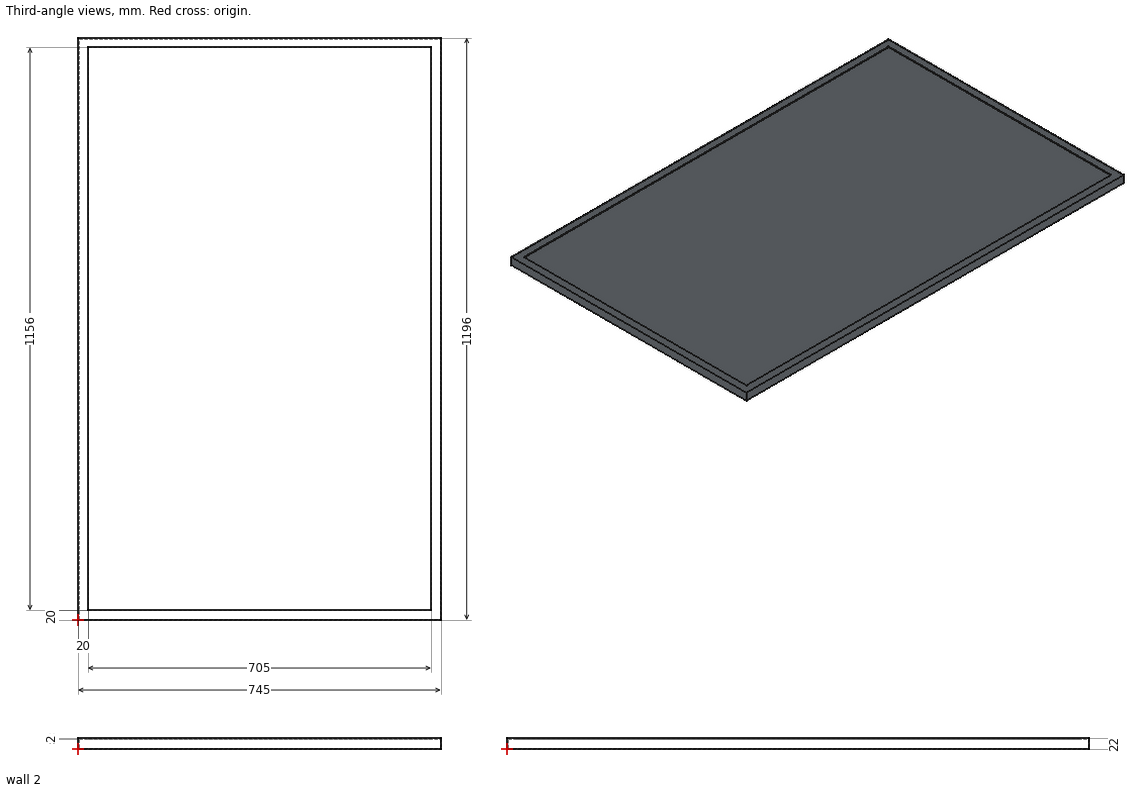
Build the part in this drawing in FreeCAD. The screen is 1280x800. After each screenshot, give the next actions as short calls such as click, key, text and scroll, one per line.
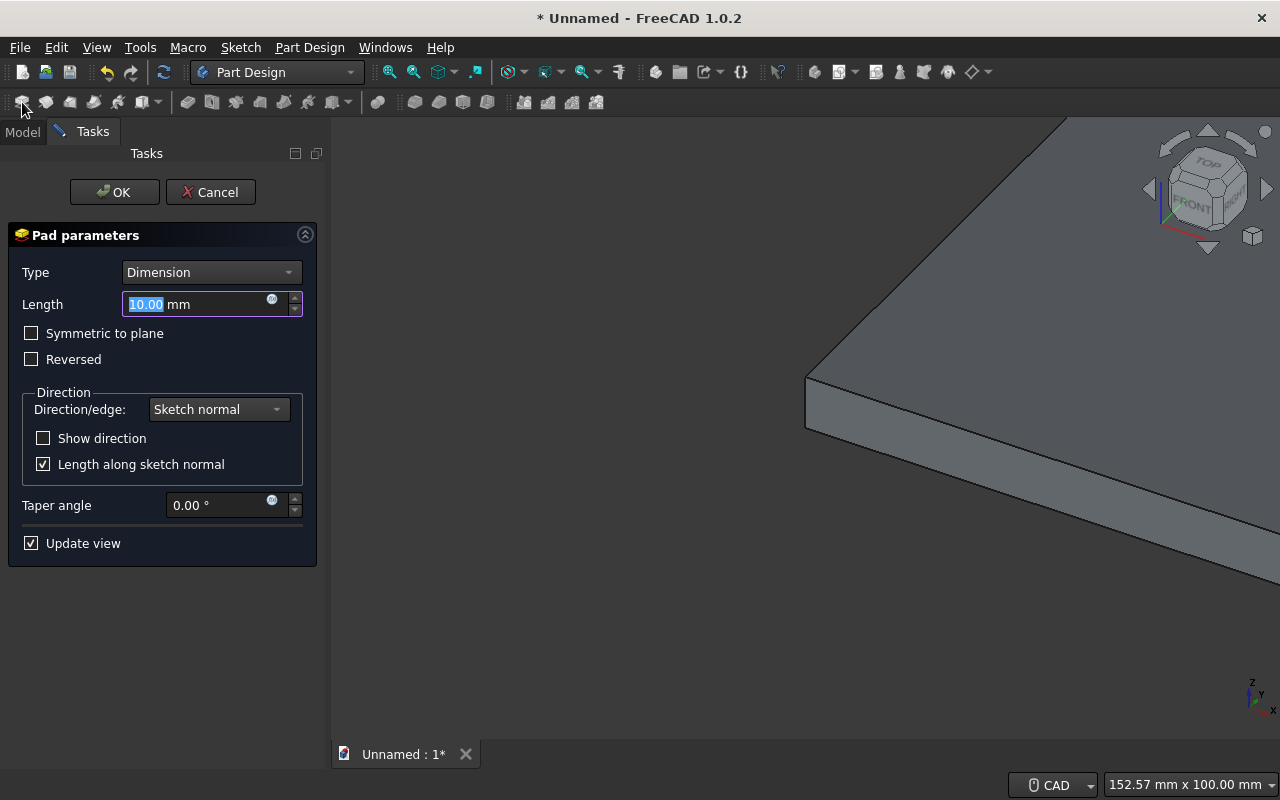
text(22)
key(Tab)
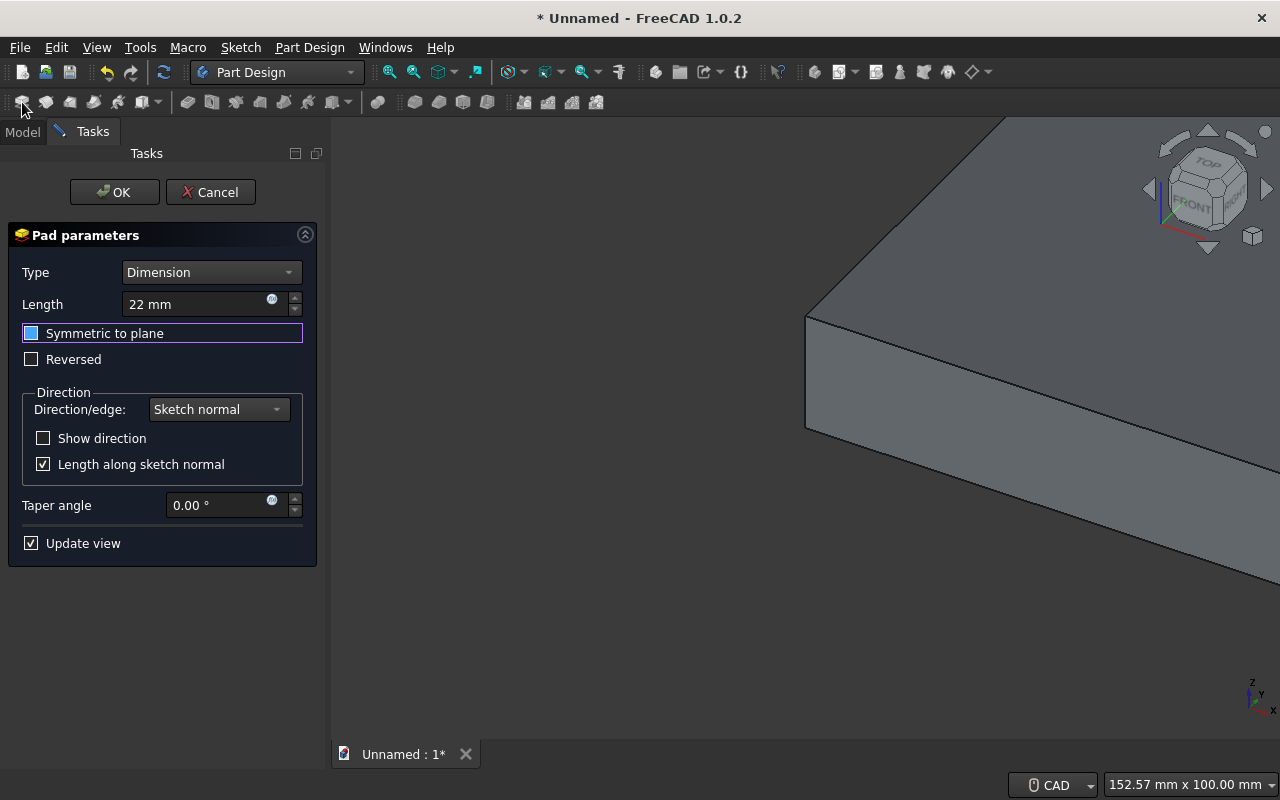
click(115, 192)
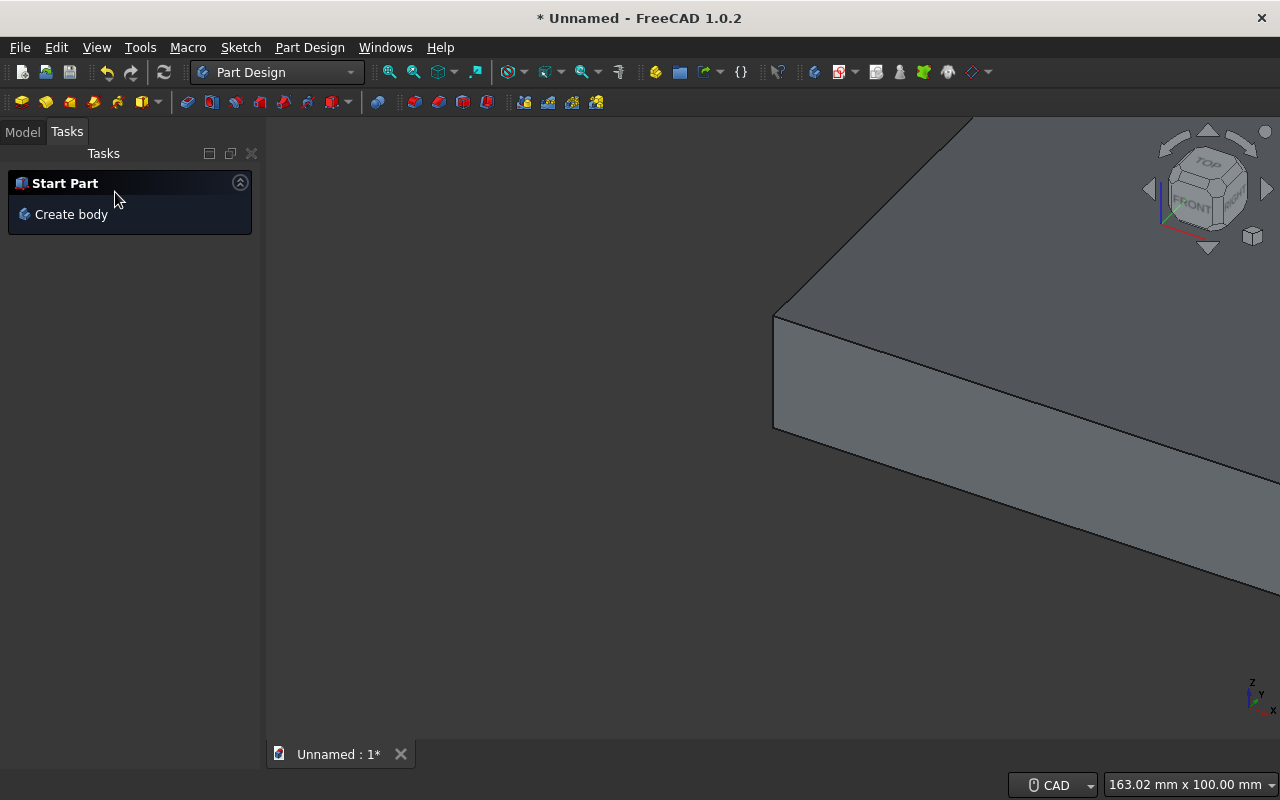
click(390, 72)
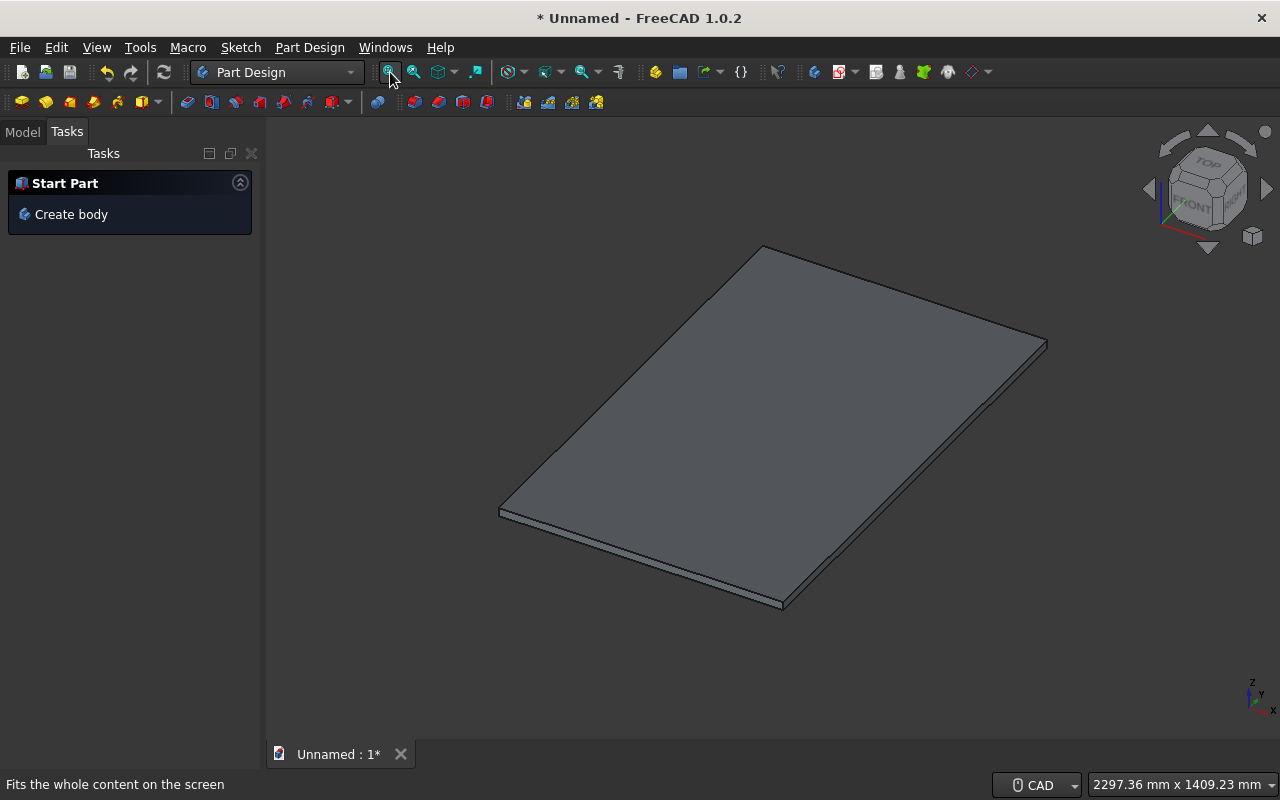
click(811, 386)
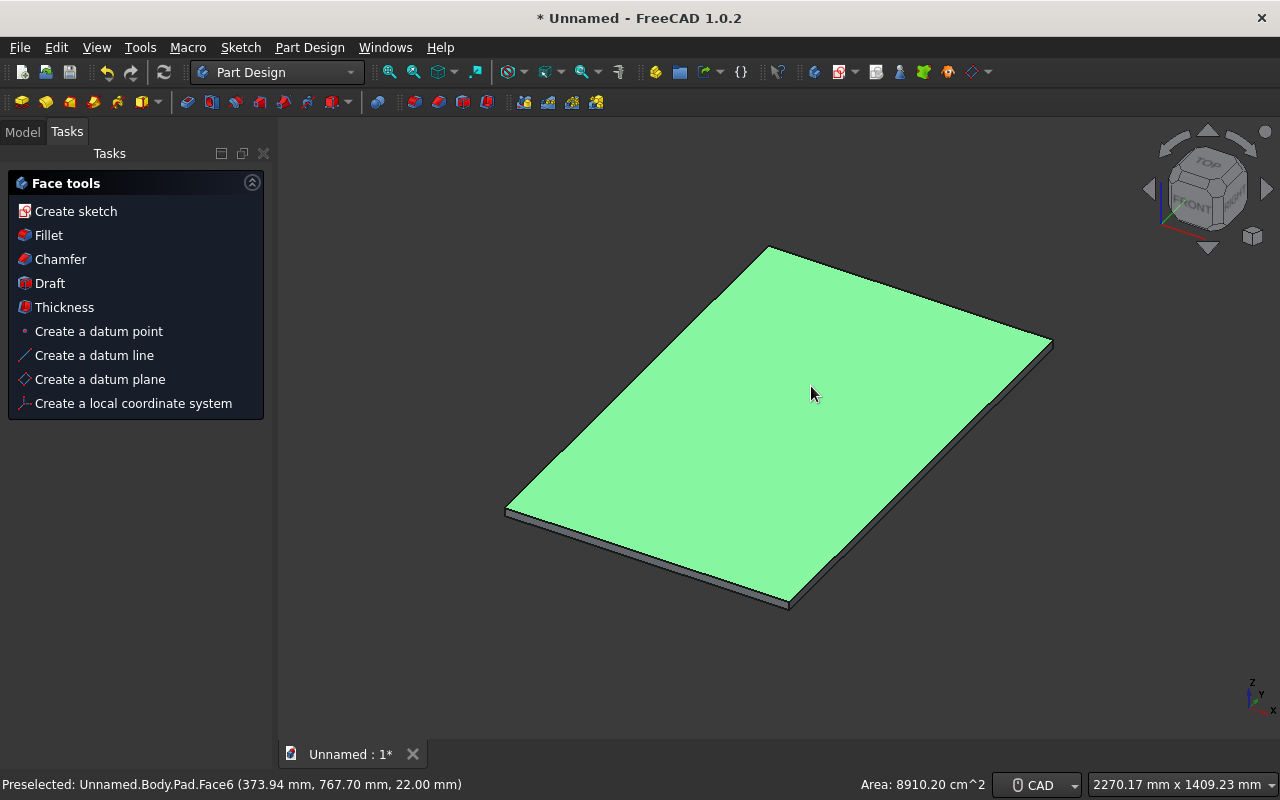
click(488, 102)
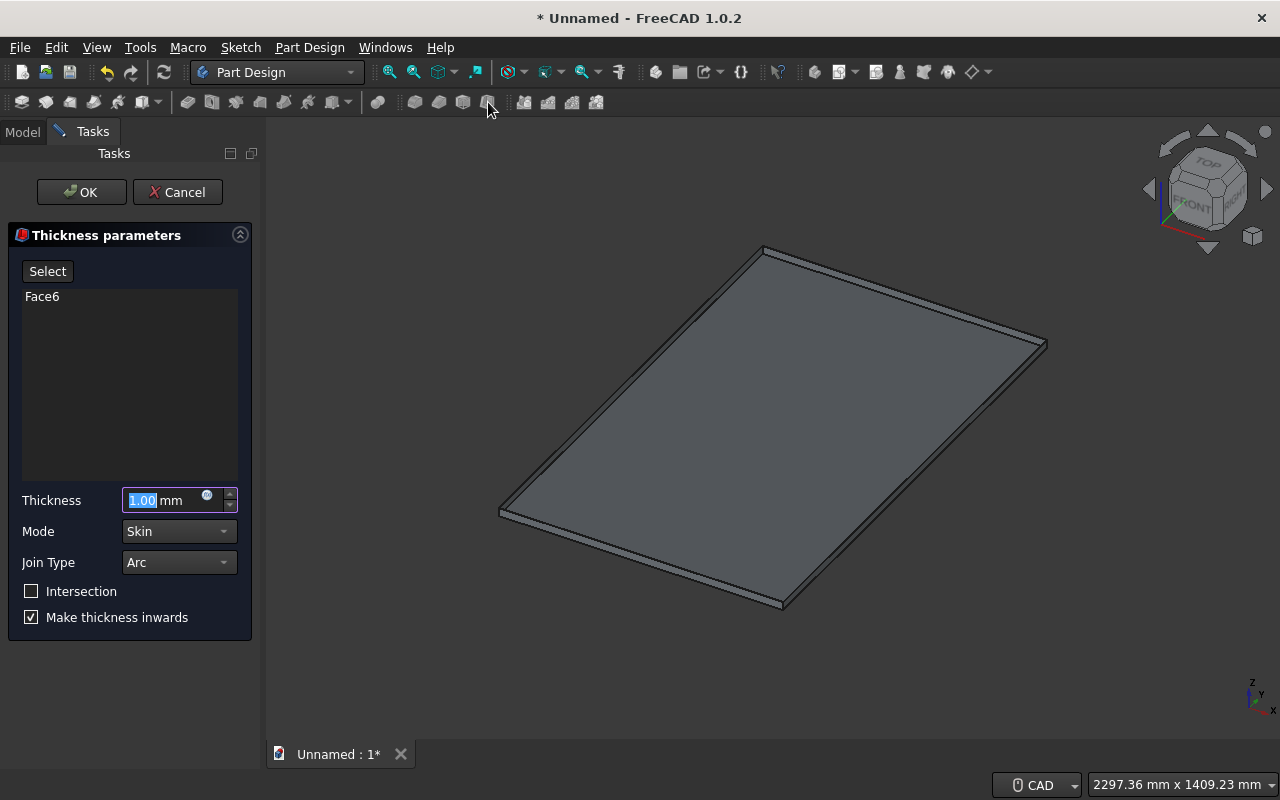
text(2)
key(Tab)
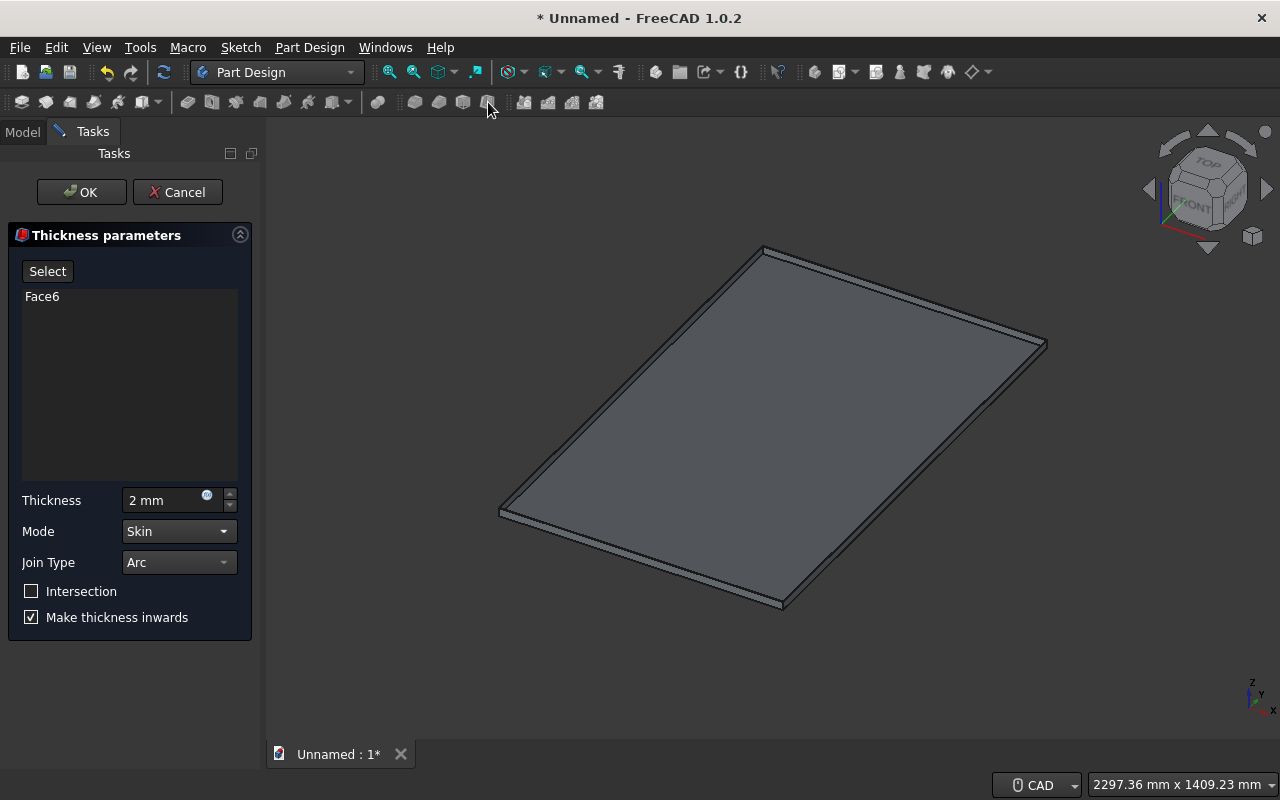
click(180, 562)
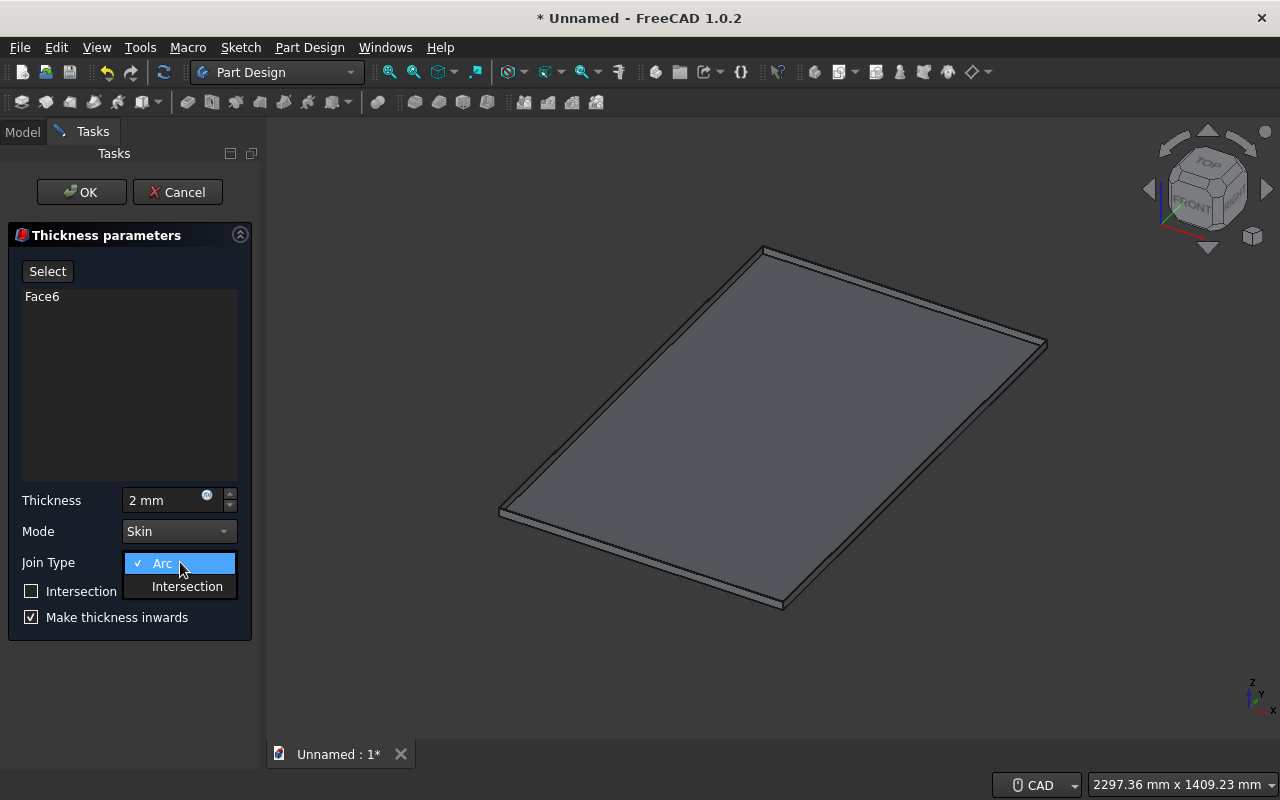
click(179, 586)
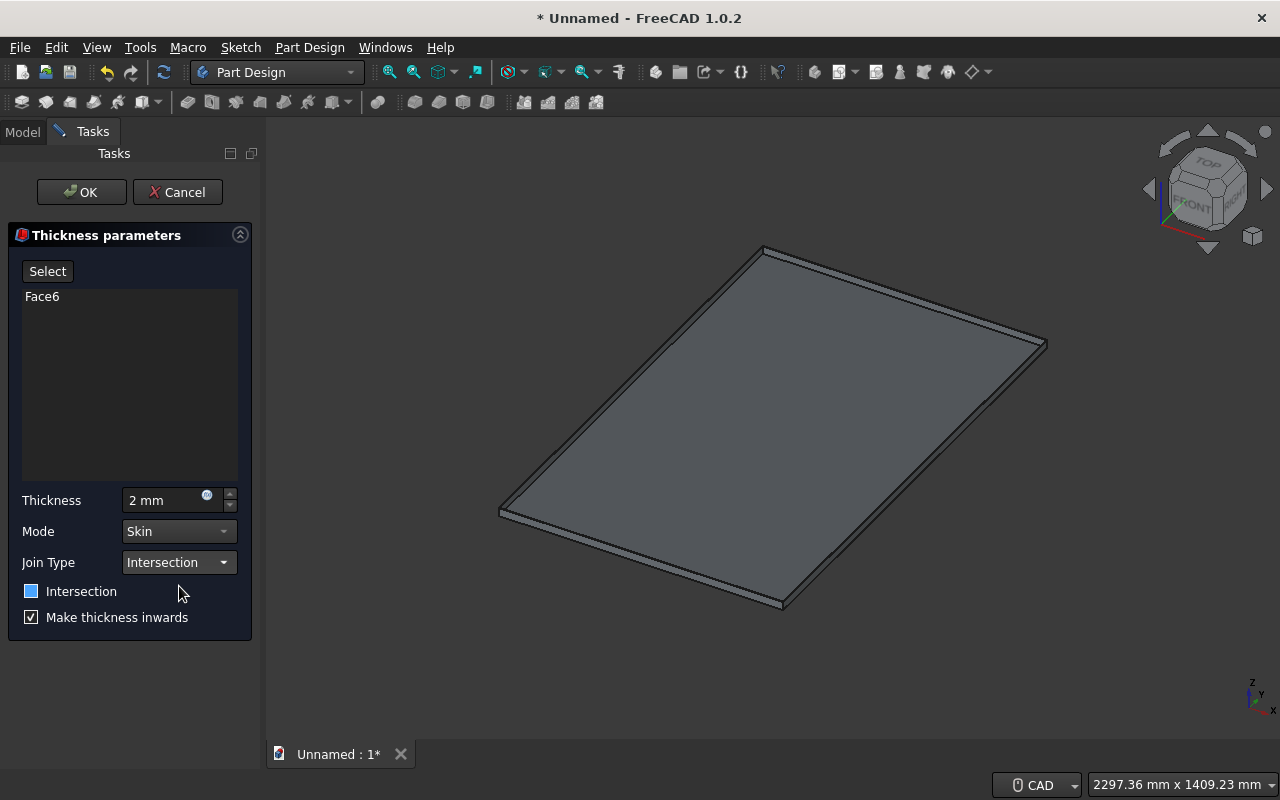
click(82, 192)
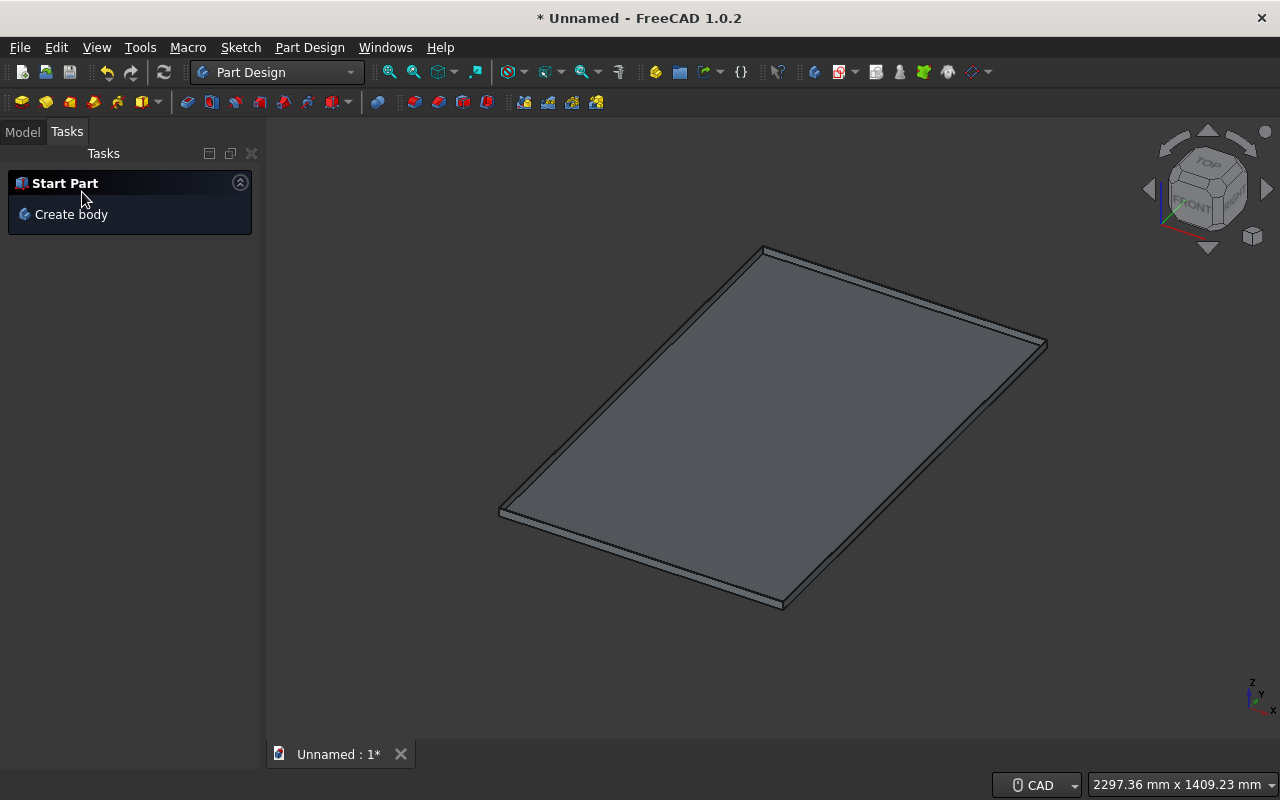
scroll(952, 308, up, 15)